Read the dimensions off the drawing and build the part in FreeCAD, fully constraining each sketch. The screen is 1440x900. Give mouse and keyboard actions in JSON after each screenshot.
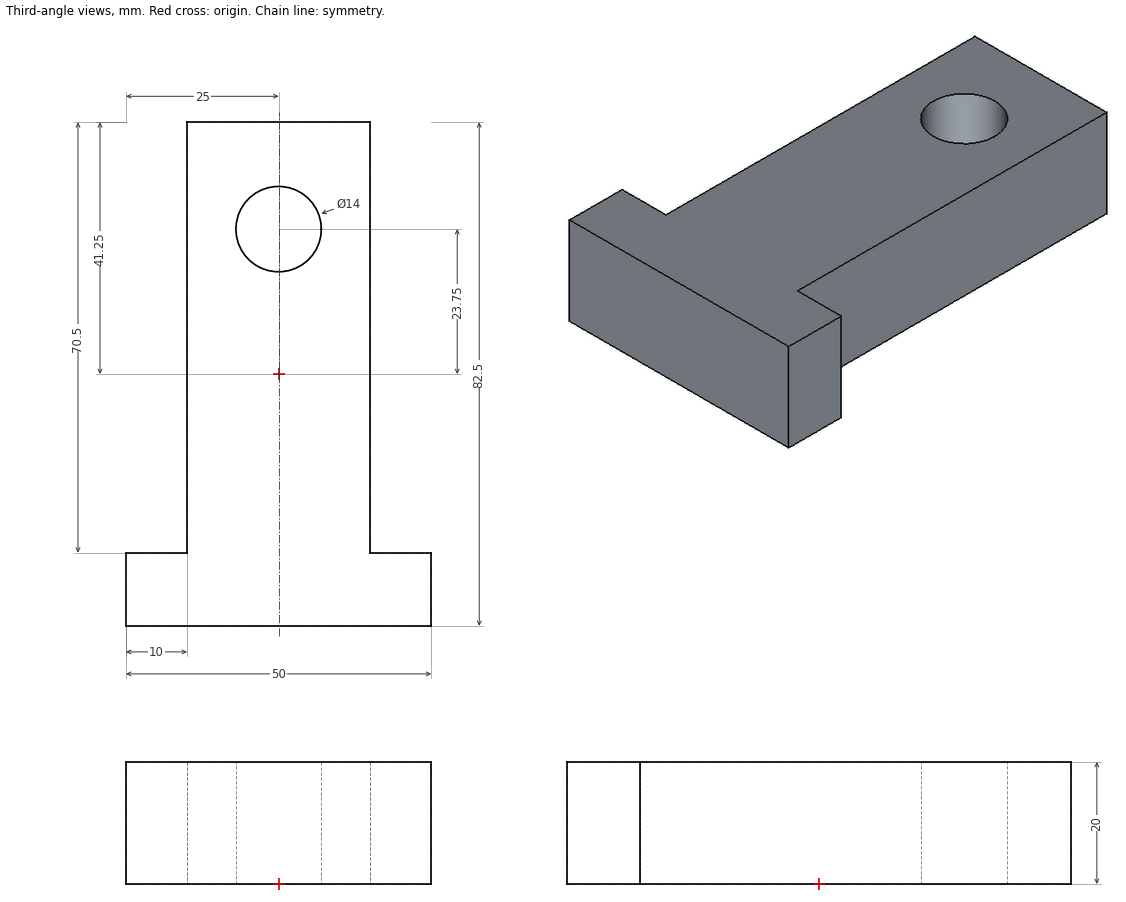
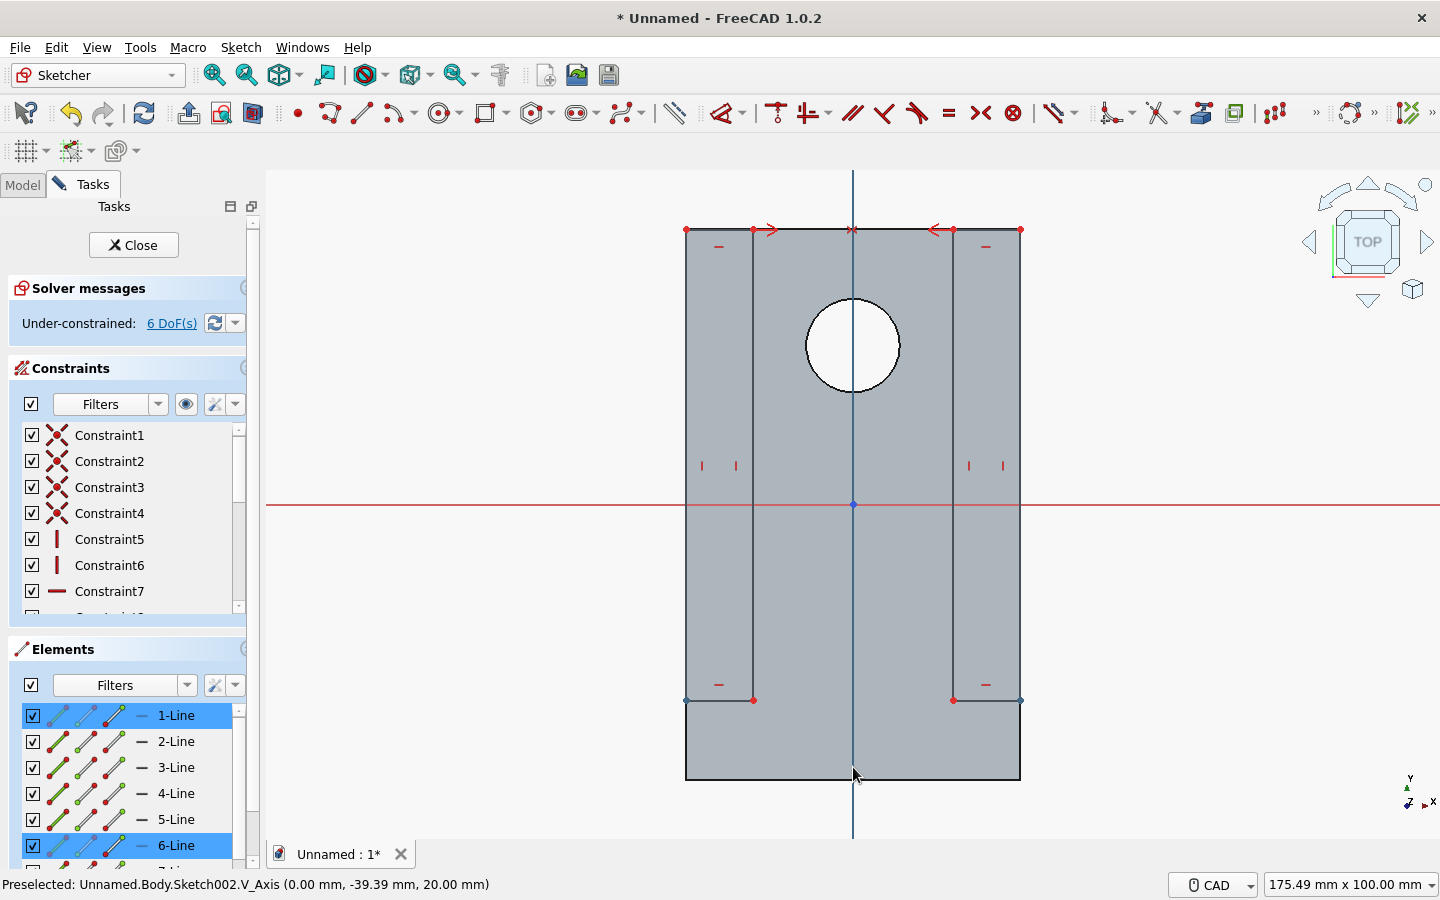
{"action": "left_click", "coordinate": [982, 114]}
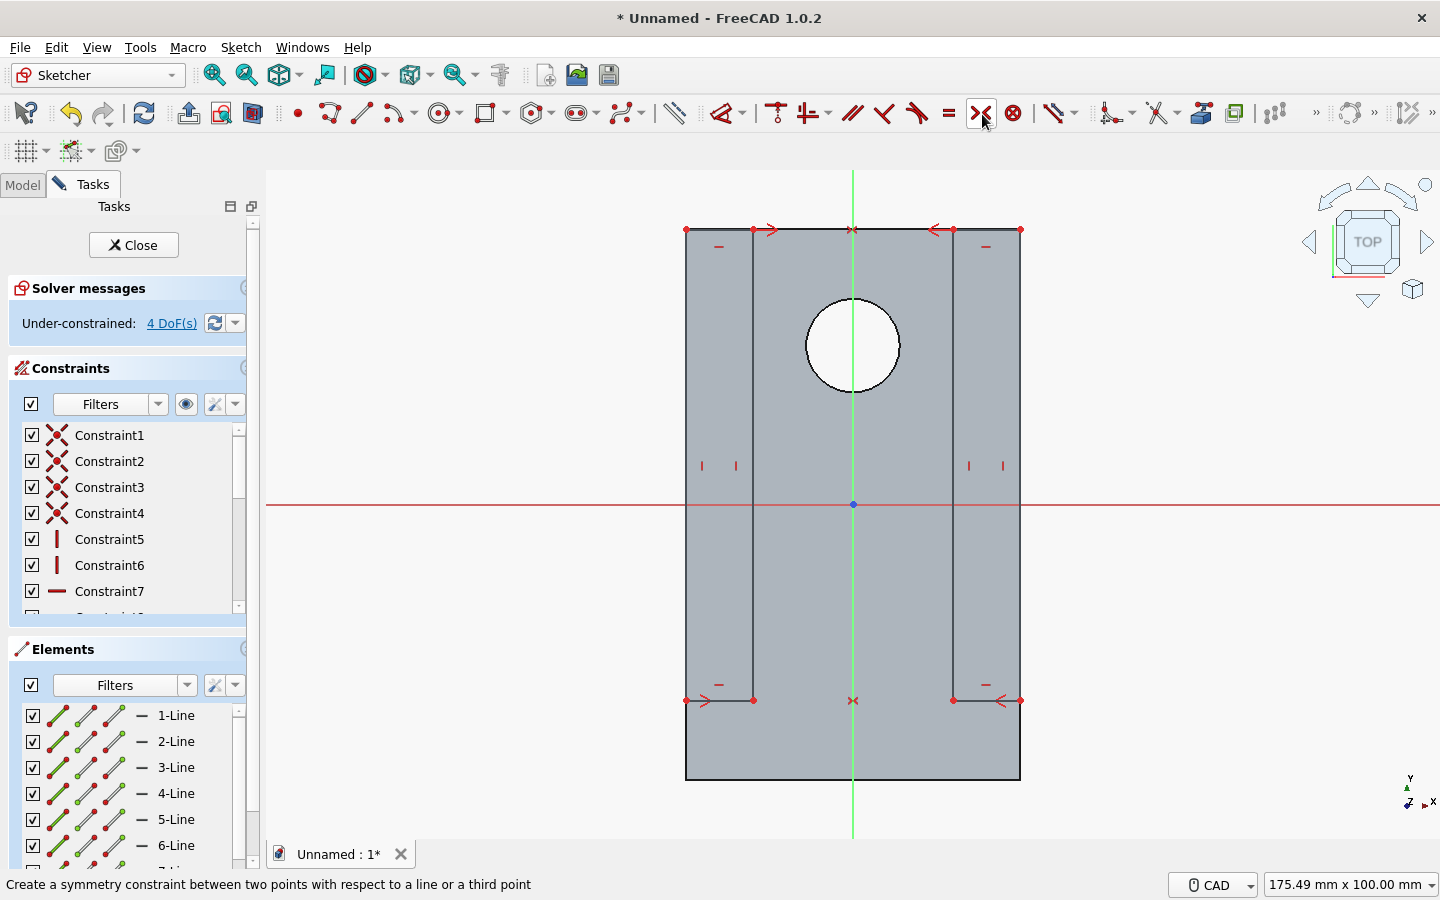
{"action": "left_click", "coordinate": [722, 114]}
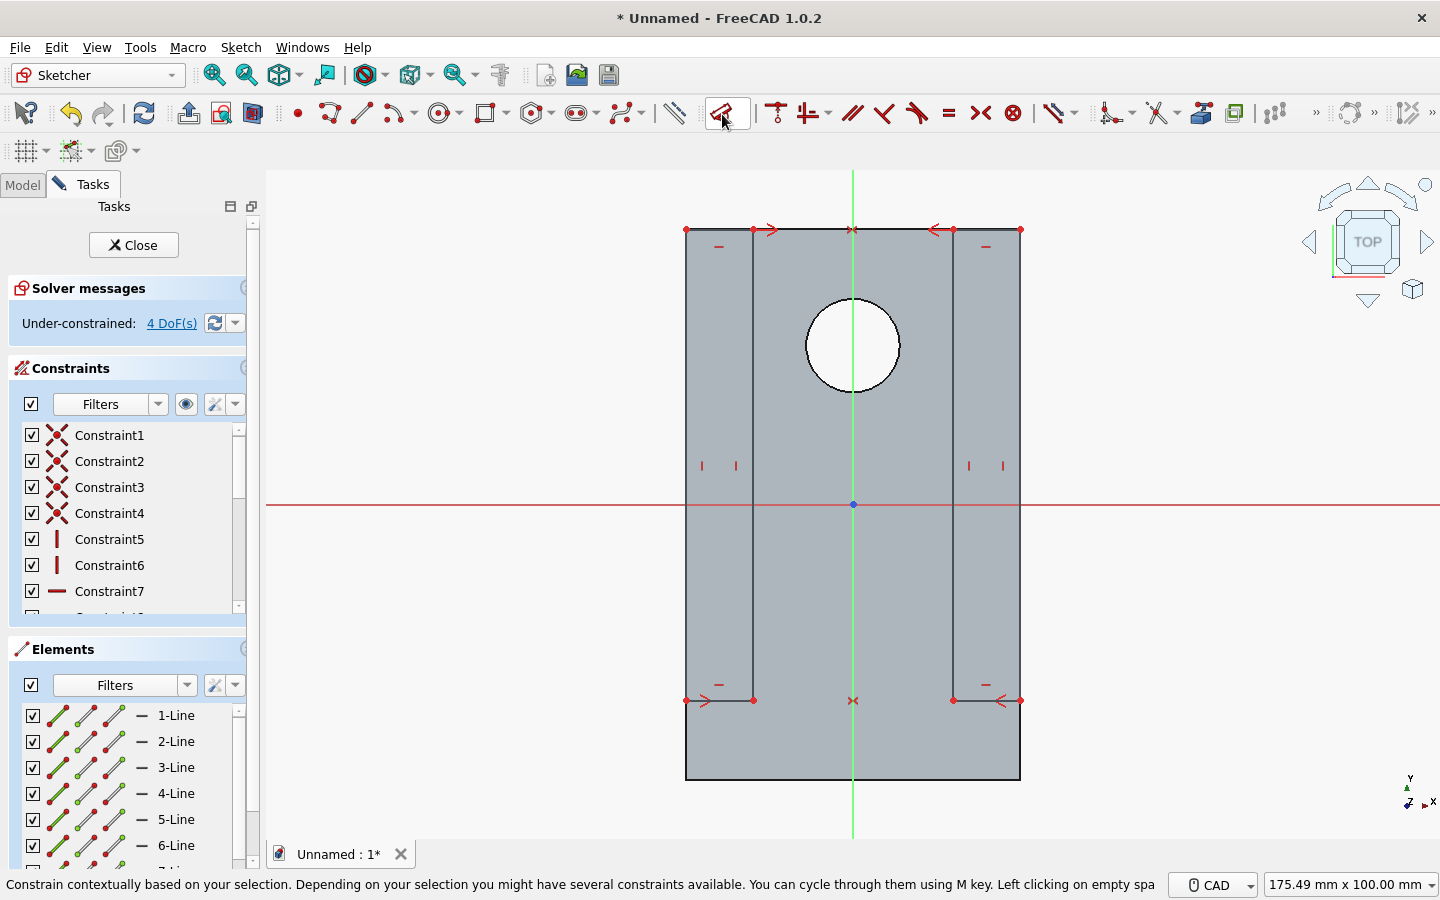
{"action": "left_click", "coordinate": [706, 701]}
{"action": "left_click", "coordinate": [720, 735]}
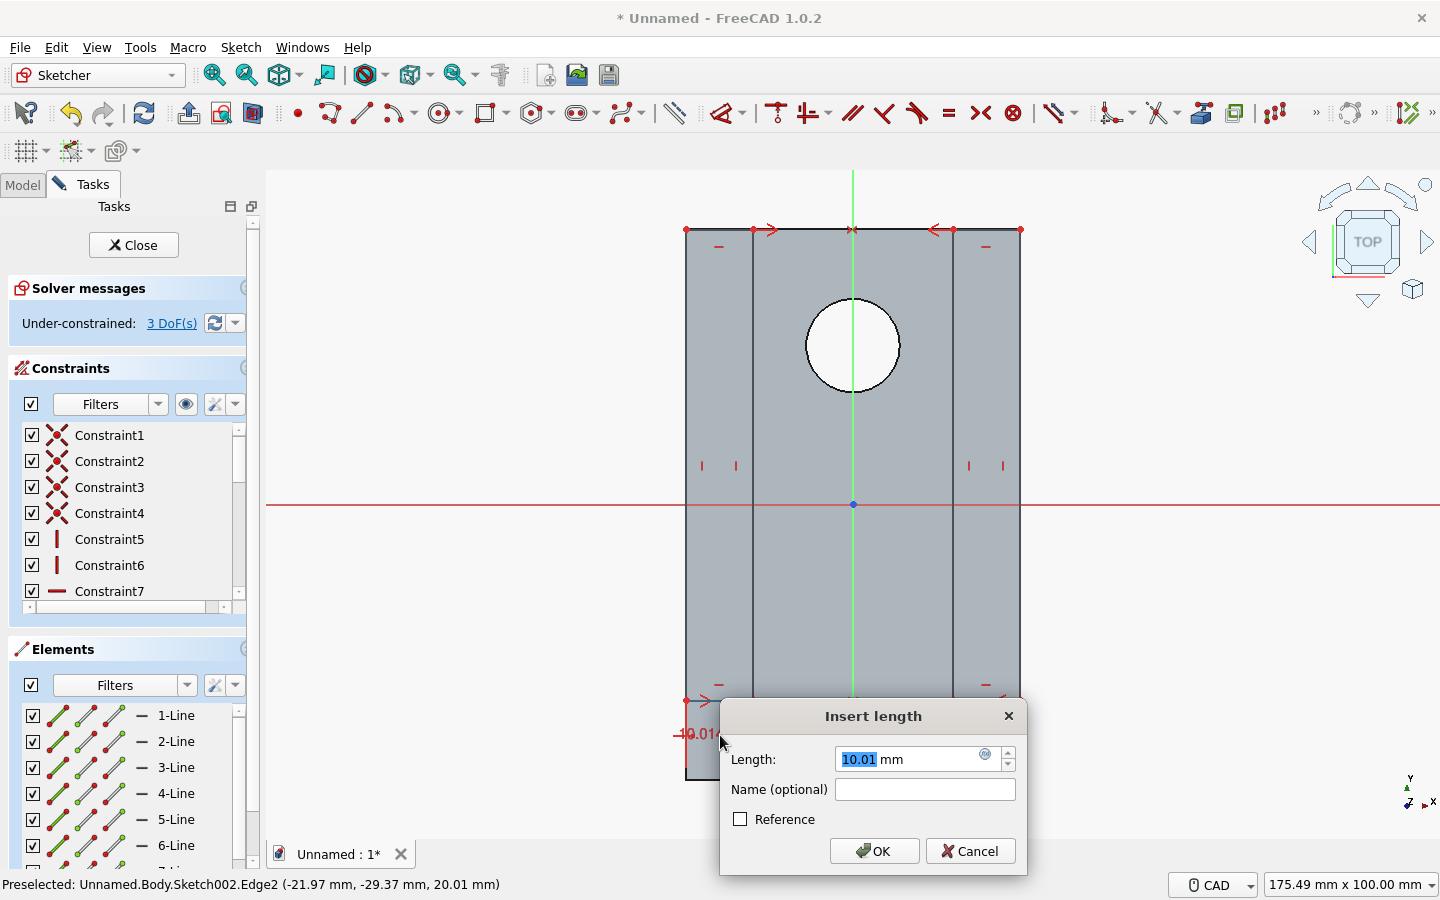
{"action": "type", "text": "10"}
{"action": "key", "text": "Return"}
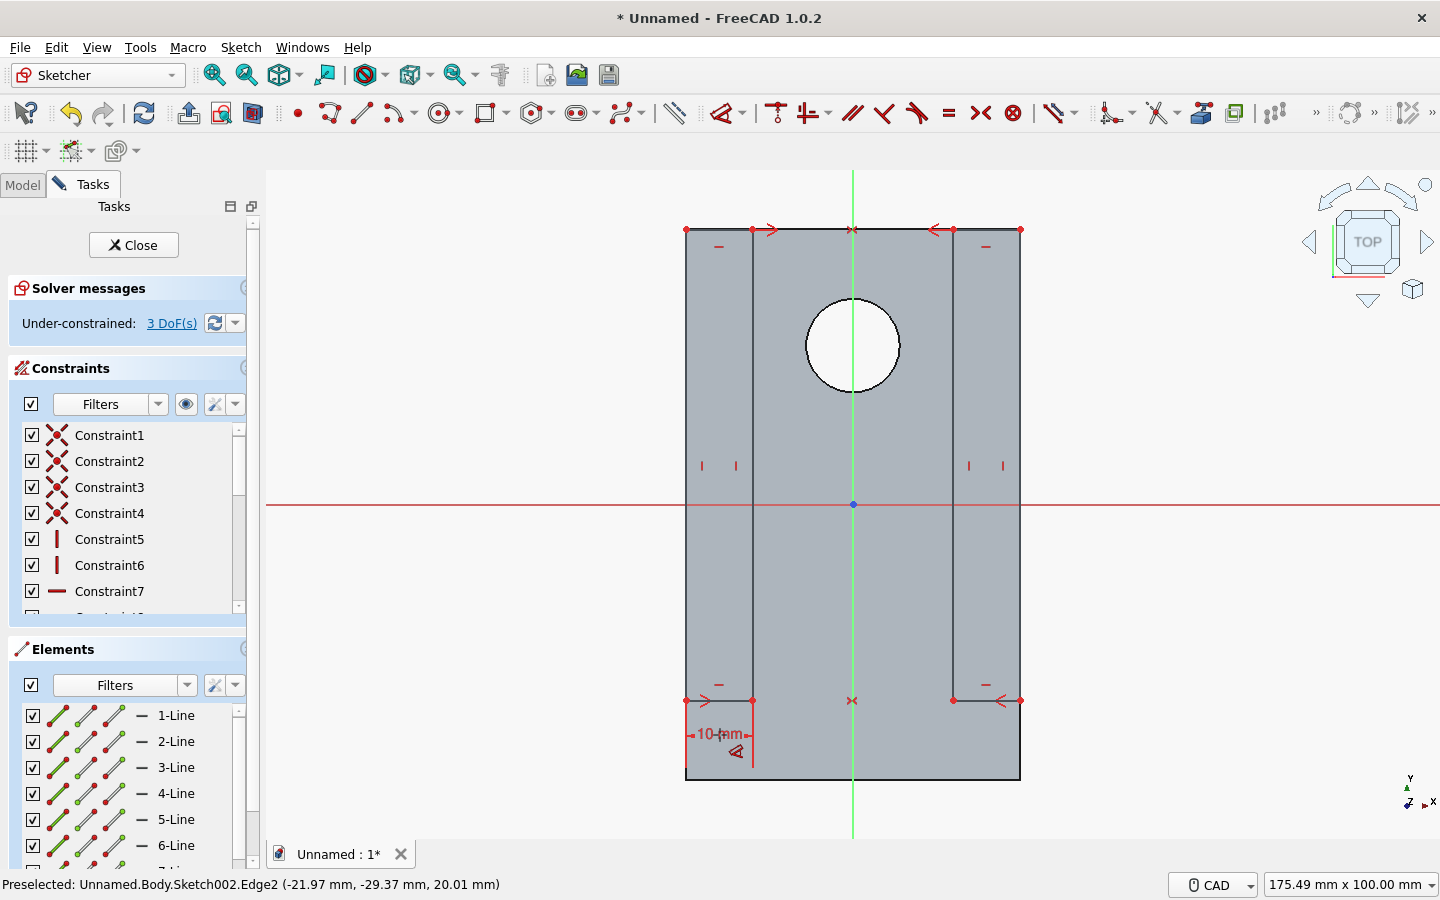
{"action": "left_click", "coordinate": [686, 230]}
{"action": "left_click", "coordinate": [769, 538]}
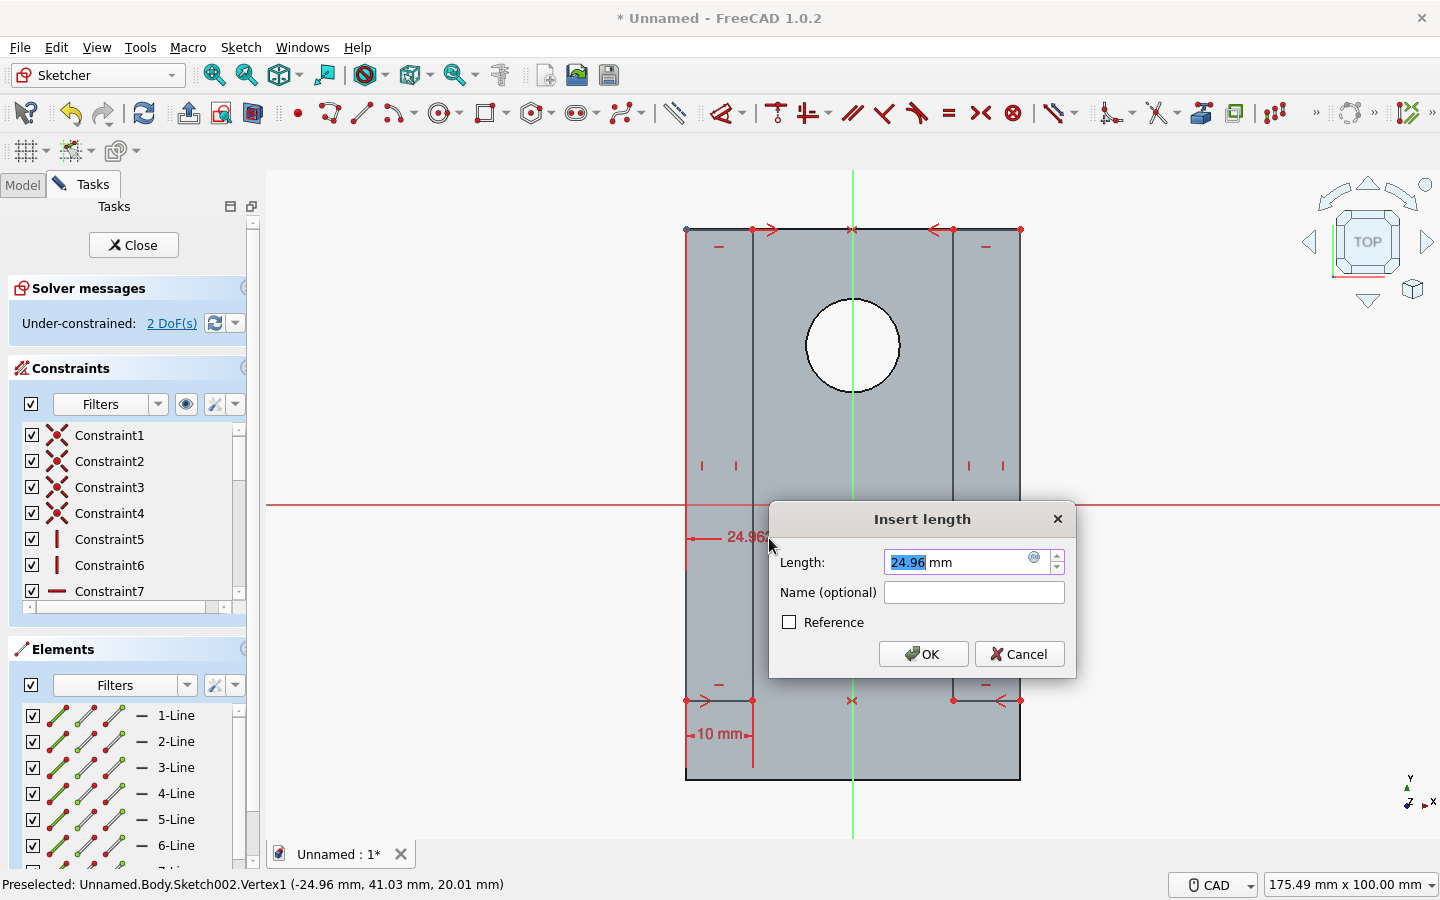
{"action": "type", "text": "25"}
{"action": "key", "text": "Return"}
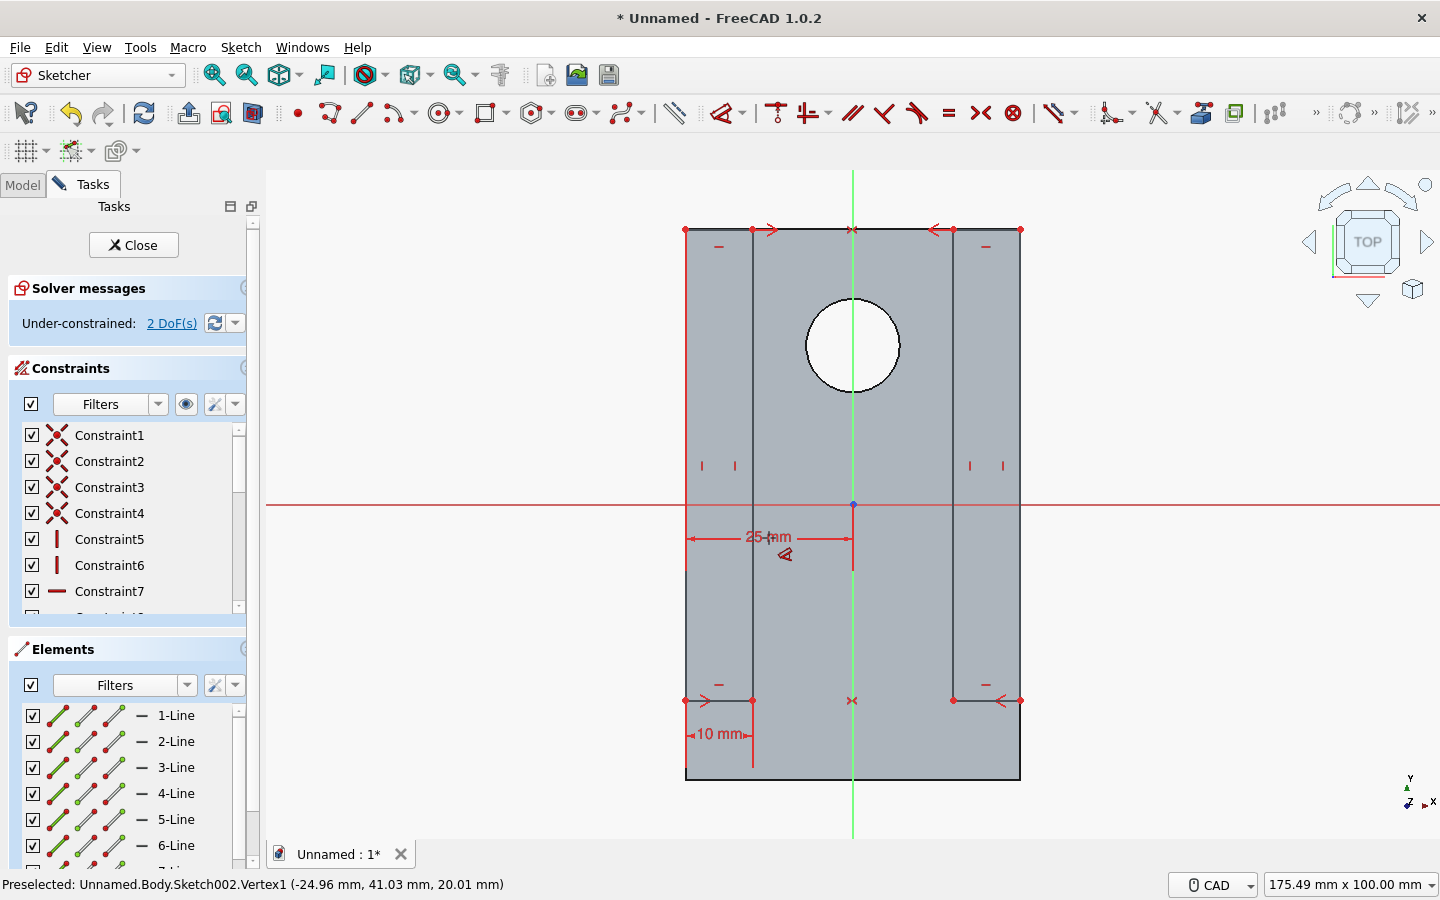
{"action": "left_click", "coordinate": [686, 371]}
{"action": "left_click", "coordinate": [652, 465]}